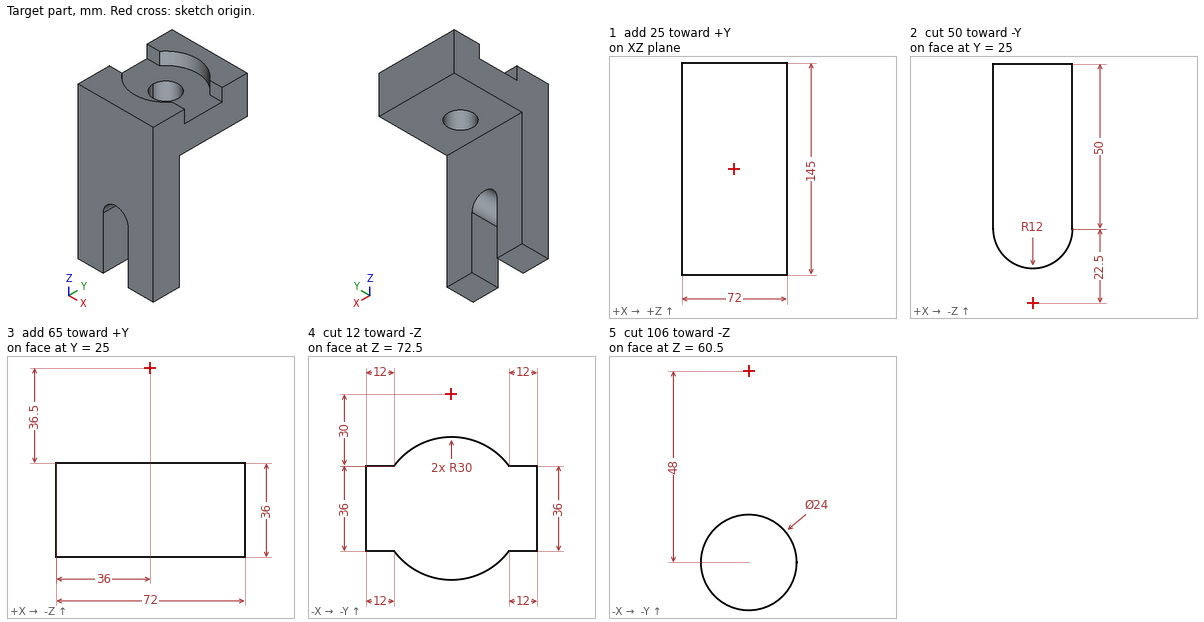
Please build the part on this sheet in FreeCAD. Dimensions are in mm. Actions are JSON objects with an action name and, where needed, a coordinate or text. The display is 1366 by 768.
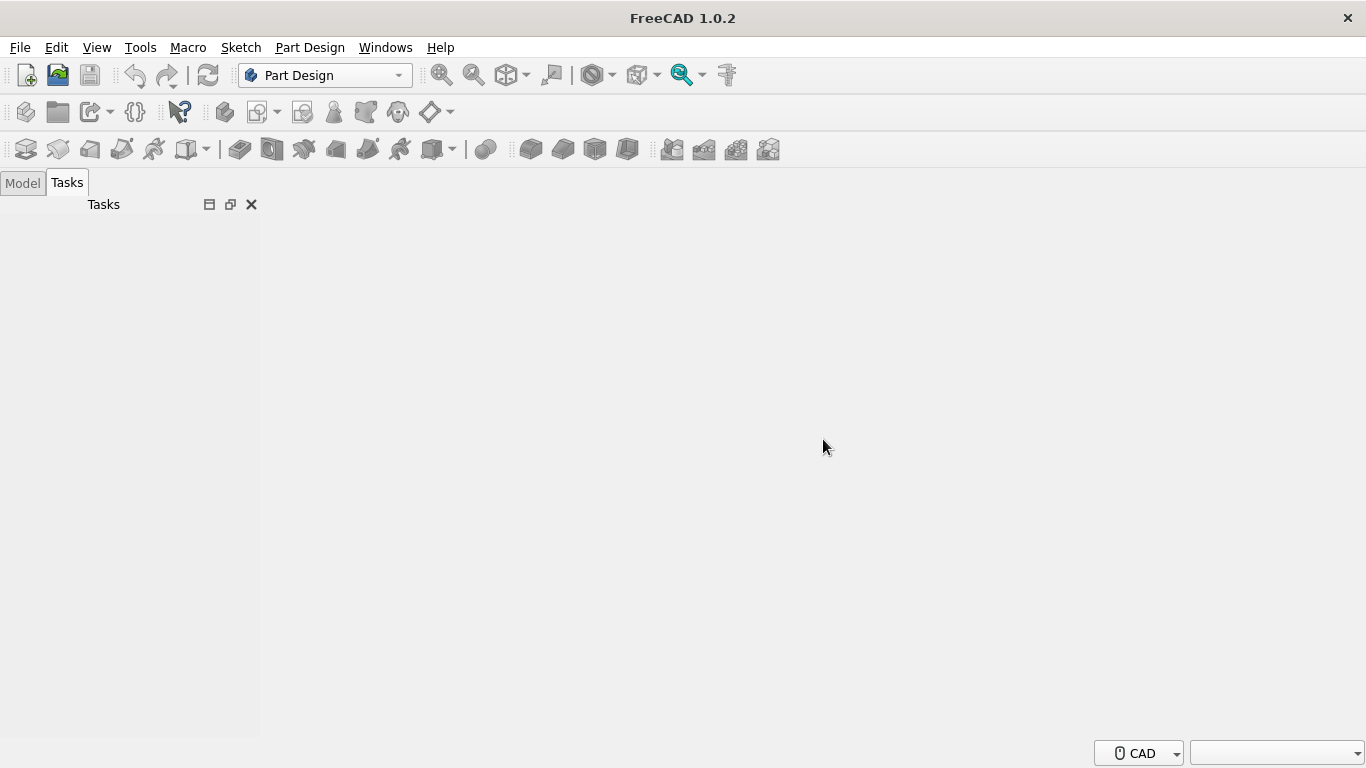
{"action": "left_click", "coordinate": [26, 76]}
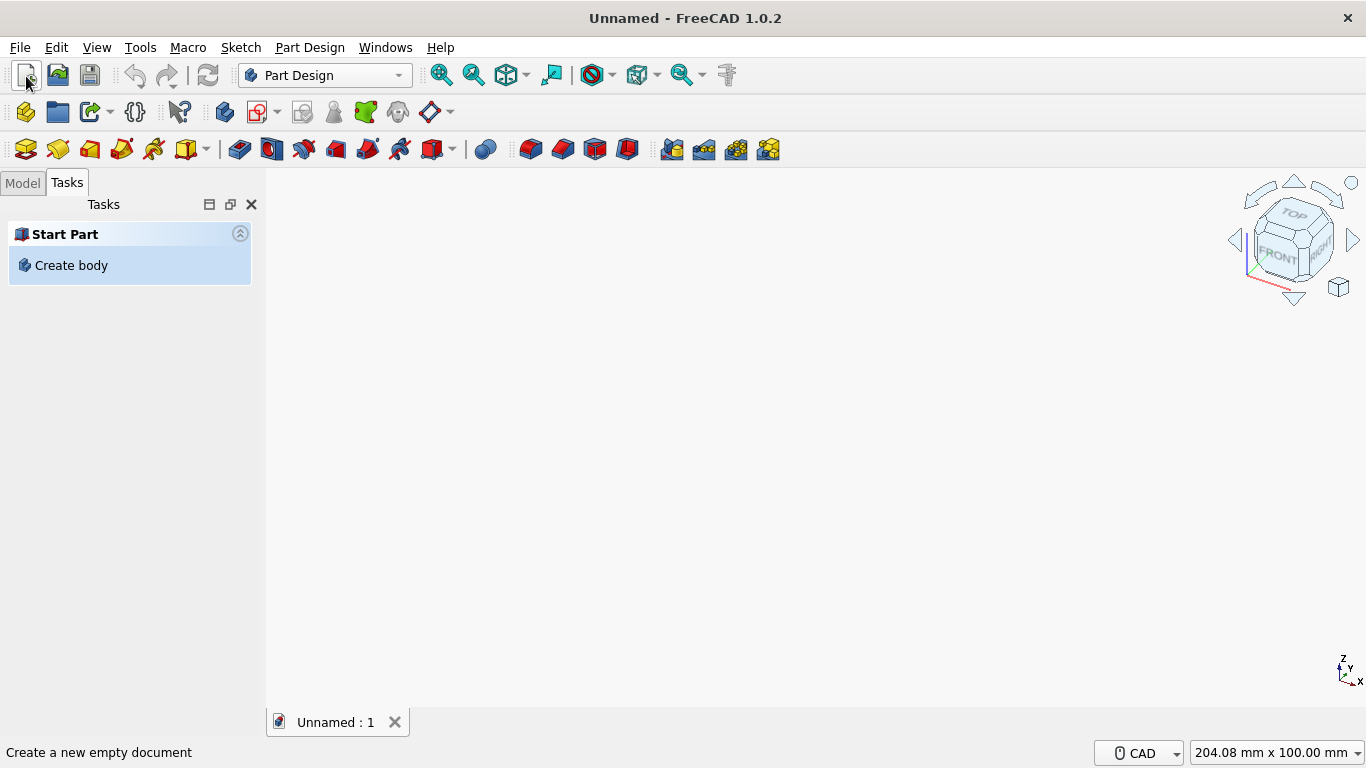
{"action": "left_click", "coordinate": [258, 112]}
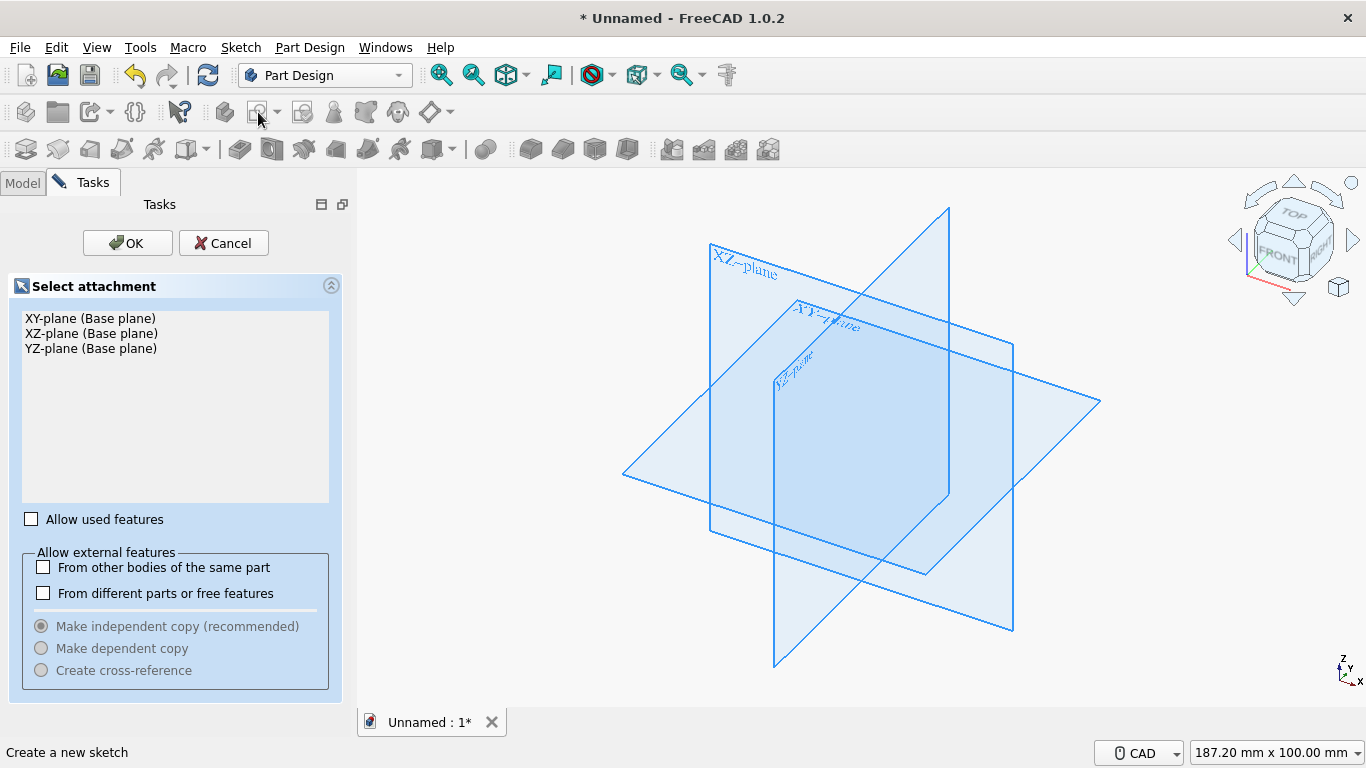
{"action": "left_click", "coordinate": [82, 334]}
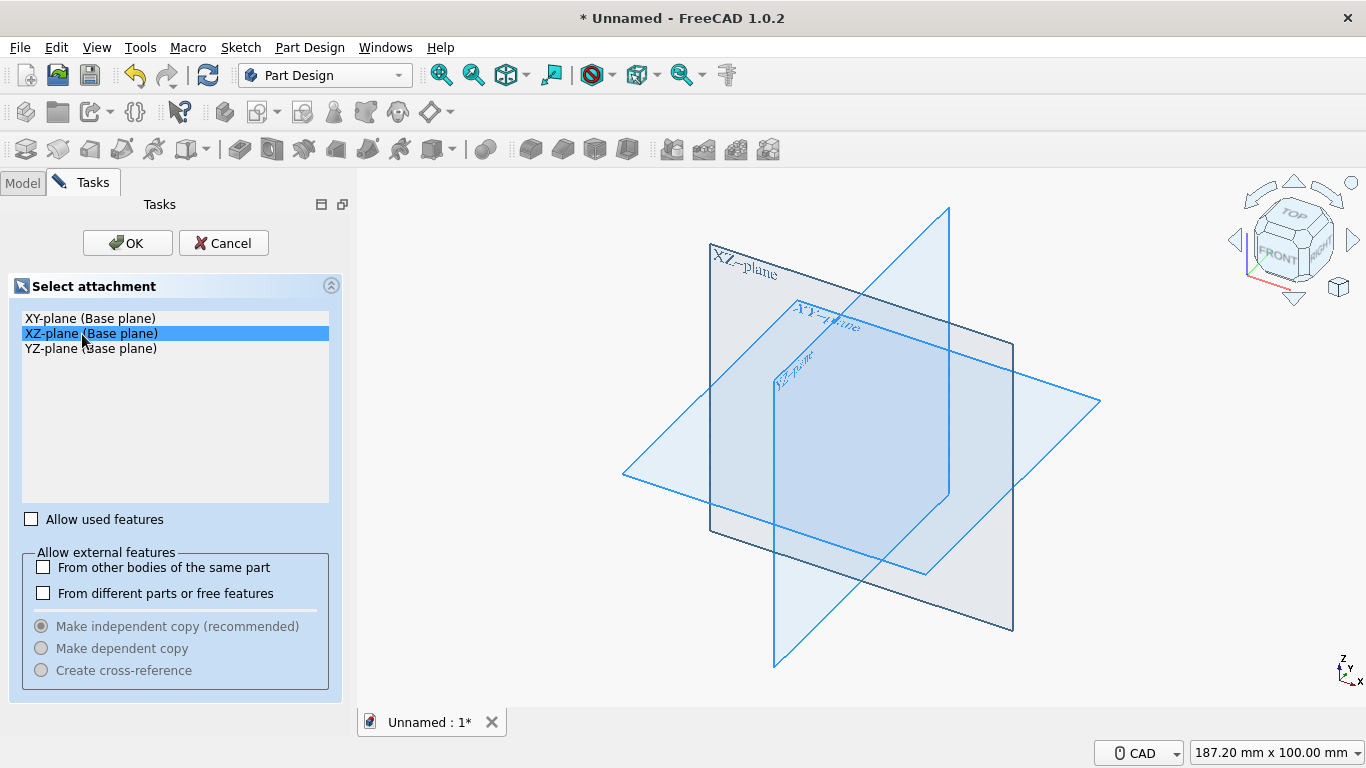
{"action": "left_click", "coordinate": [128, 243]}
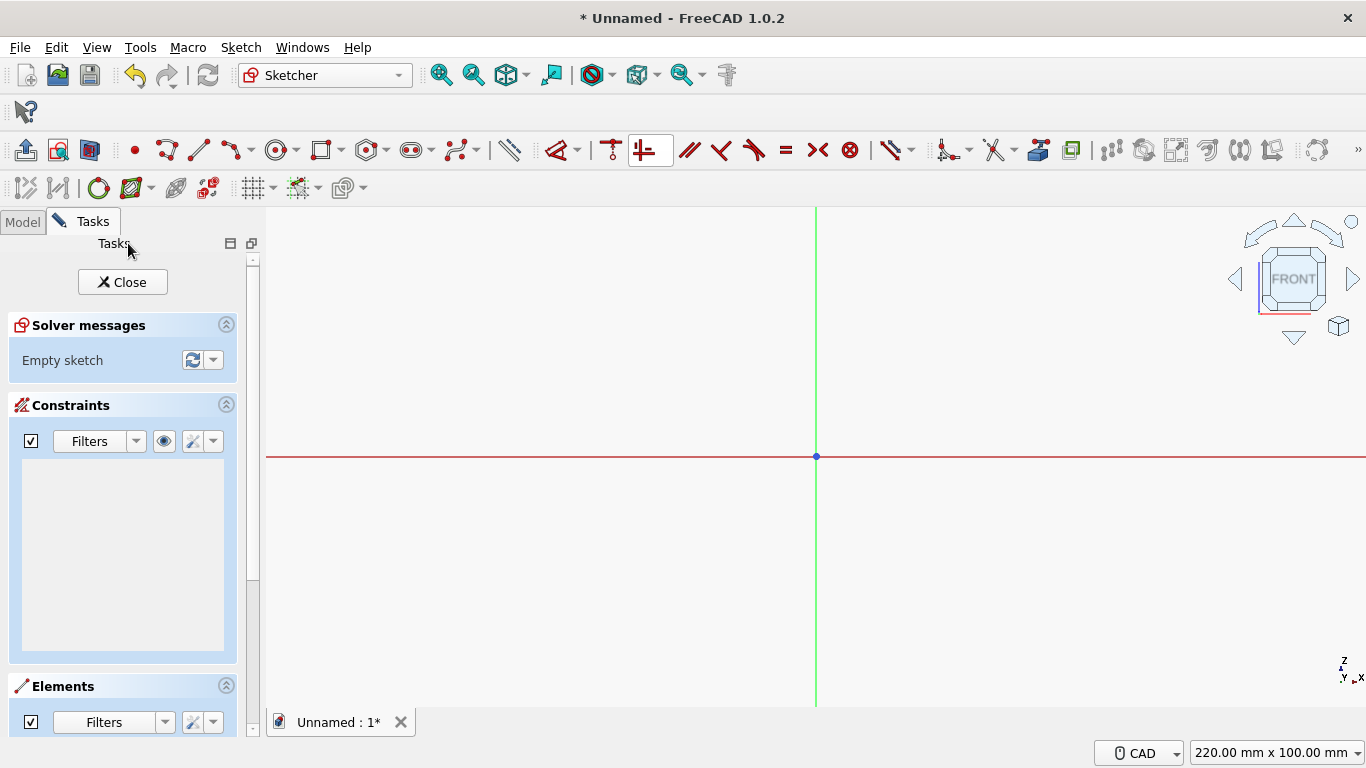
{"action": "scroll", "coordinate": [692, 457], "scroll_direction": "down", "scroll_amount": 4}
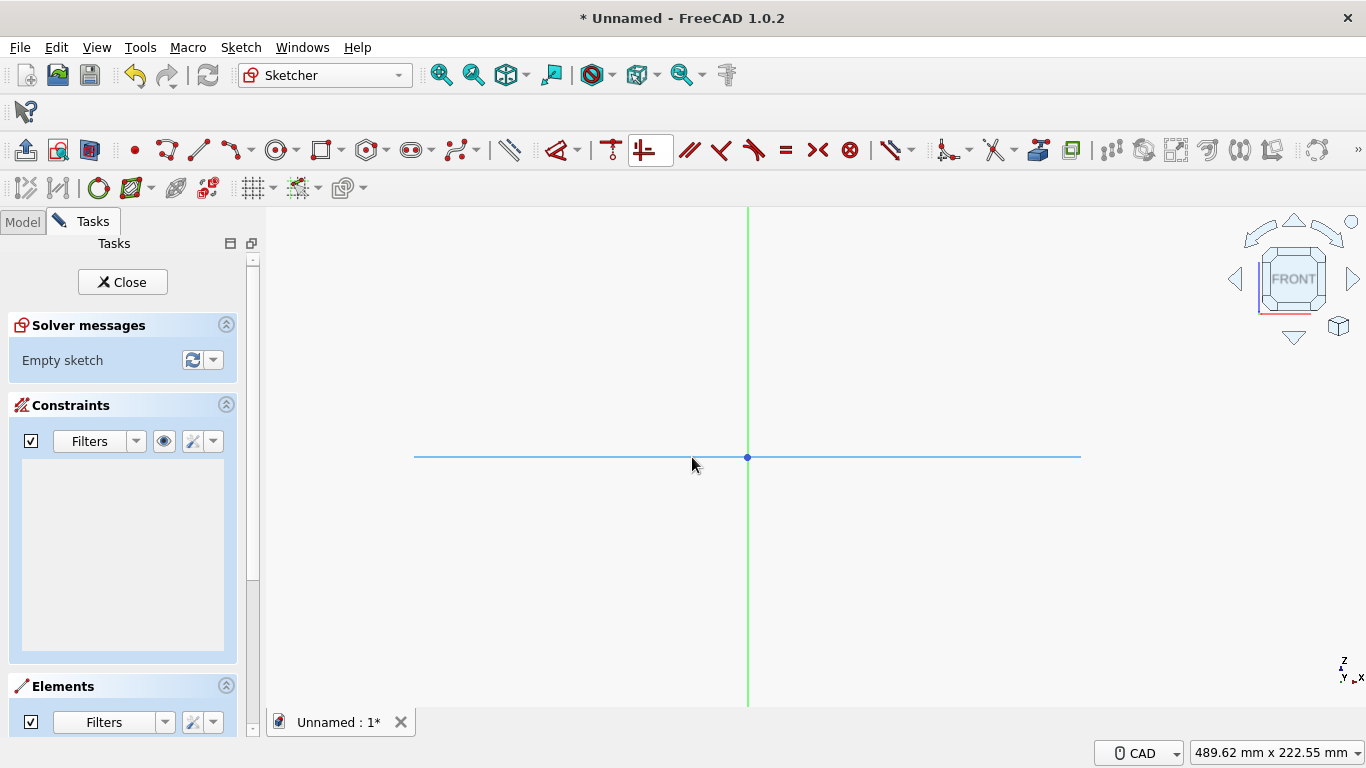
{"action": "key", "text": "g v"}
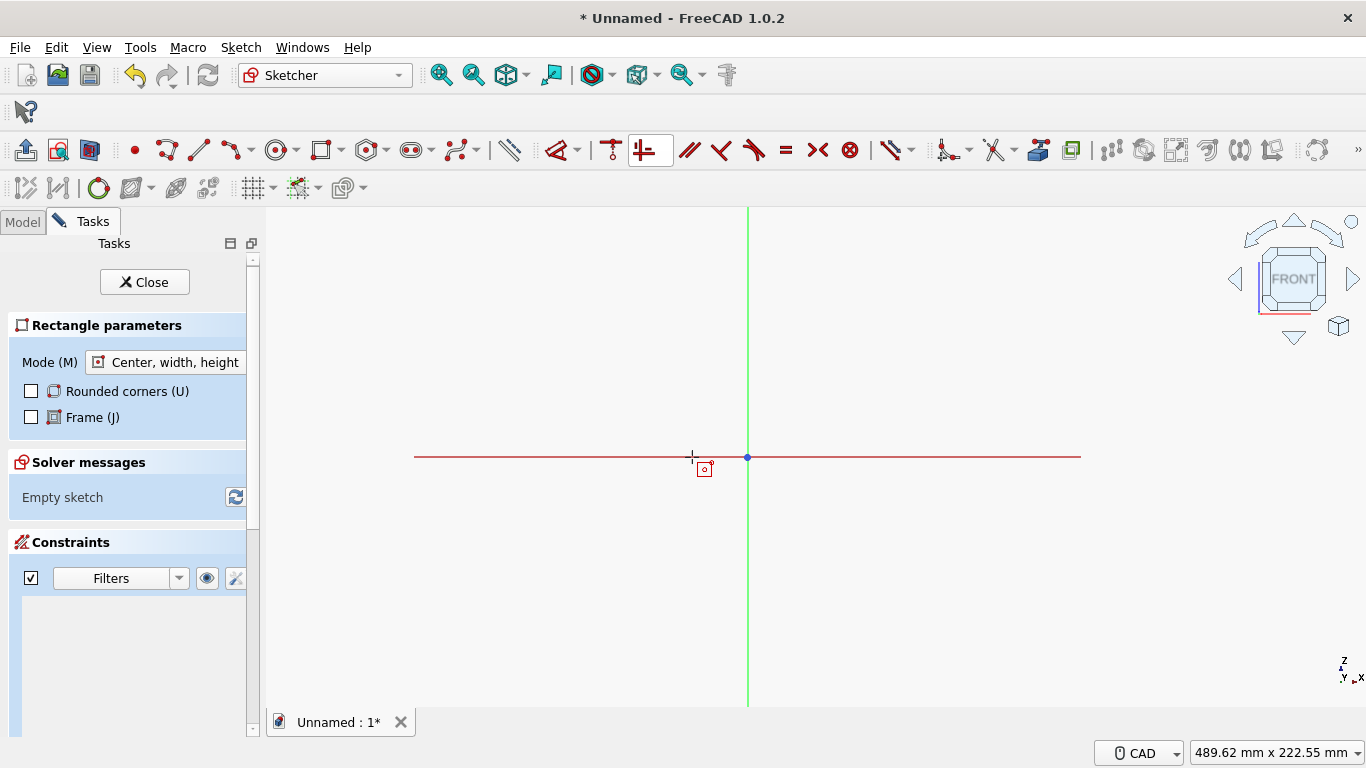
{"action": "left_click", "coordinate": [748, 457]}
{"action": "mouse_move", "coordinate": [829, 294]}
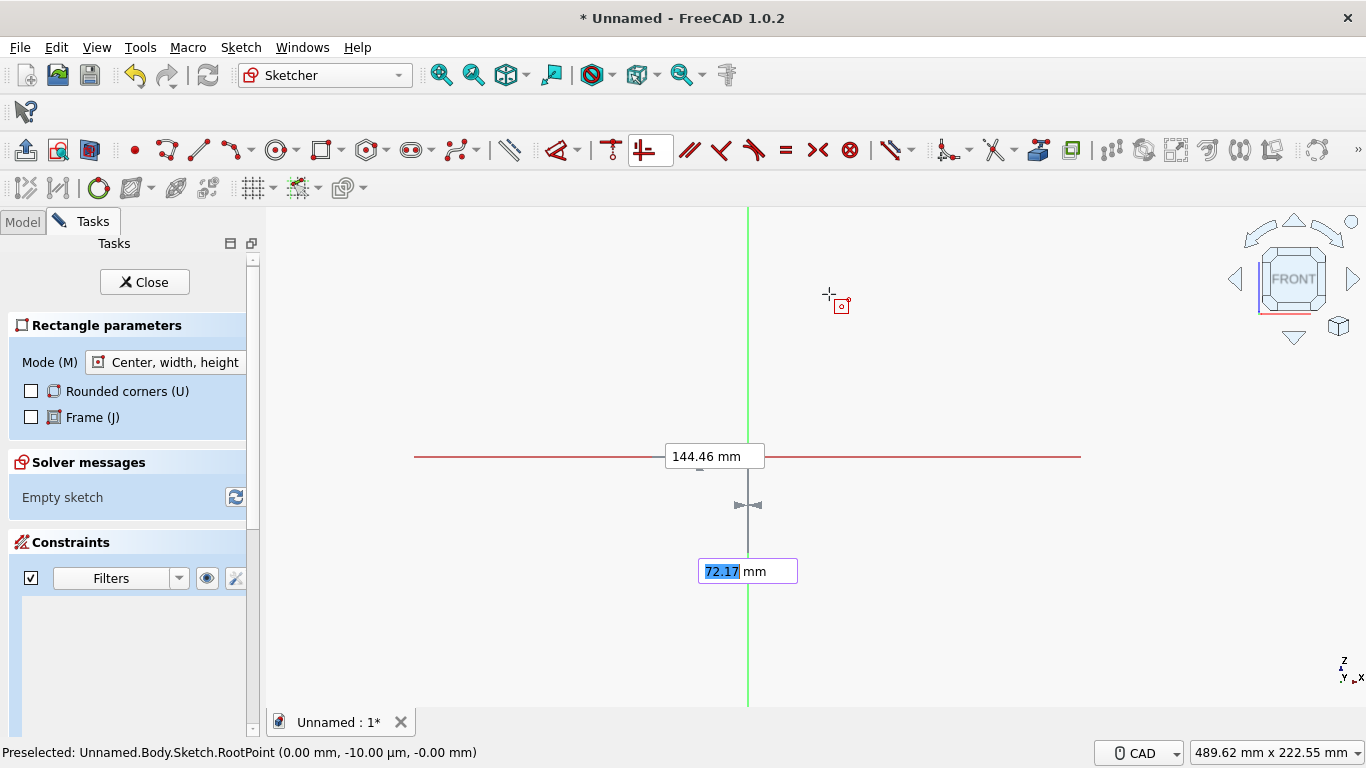
{"action": "type", "text": "72"}
{"action": "key", "text": "Tab"}
{"action": "type", "text": "145"}
{"action": "key", "text": "Return"}
{"action": "key", "text": "Escape"}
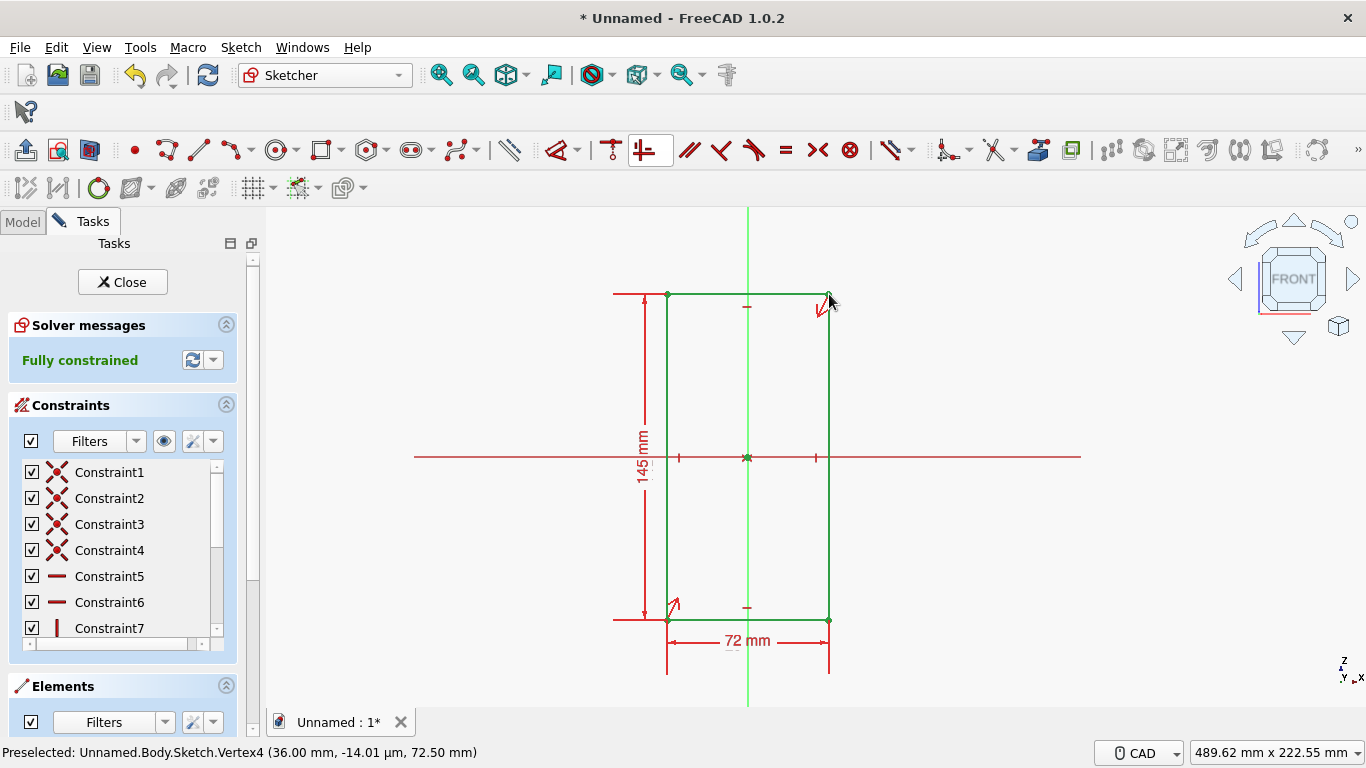
{"action": "left_click", "coordinate": [123, 282]}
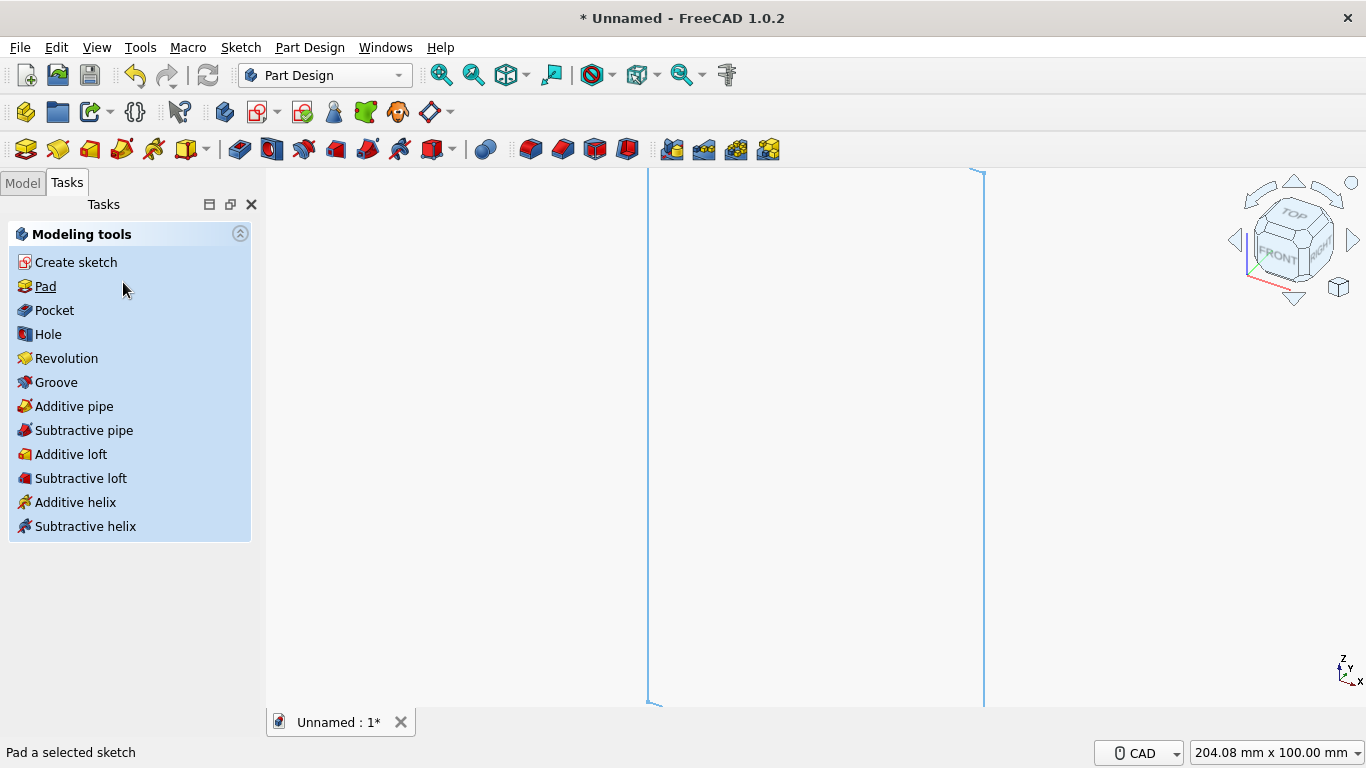
{"action": "left_click", "coordinate": [26, 150]}